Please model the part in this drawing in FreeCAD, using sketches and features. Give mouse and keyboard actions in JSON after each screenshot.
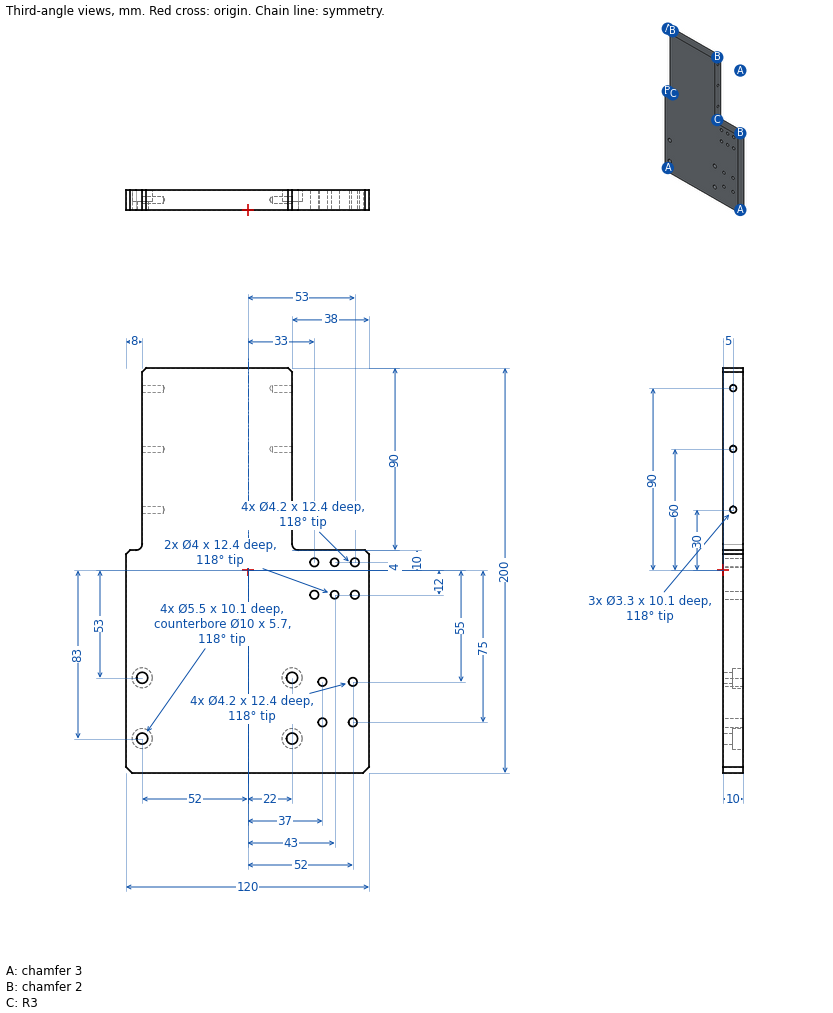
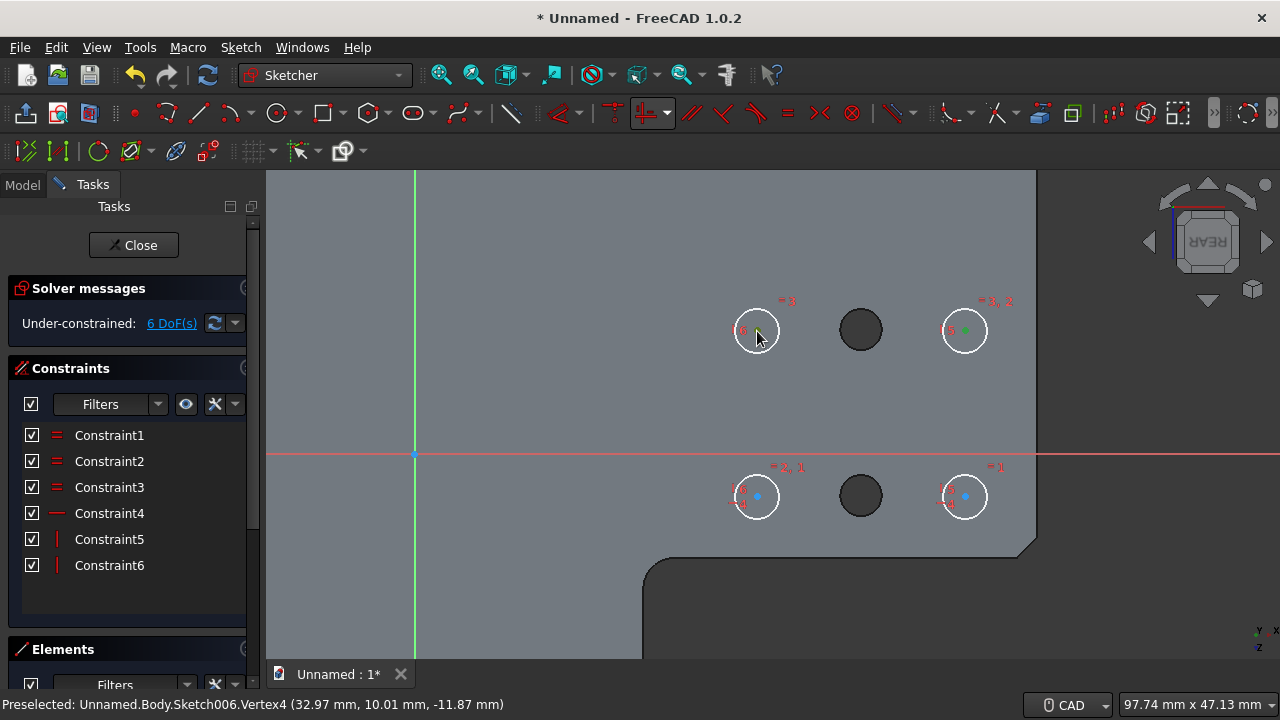
{"action": "left_click", "coordinate": [670, 114]}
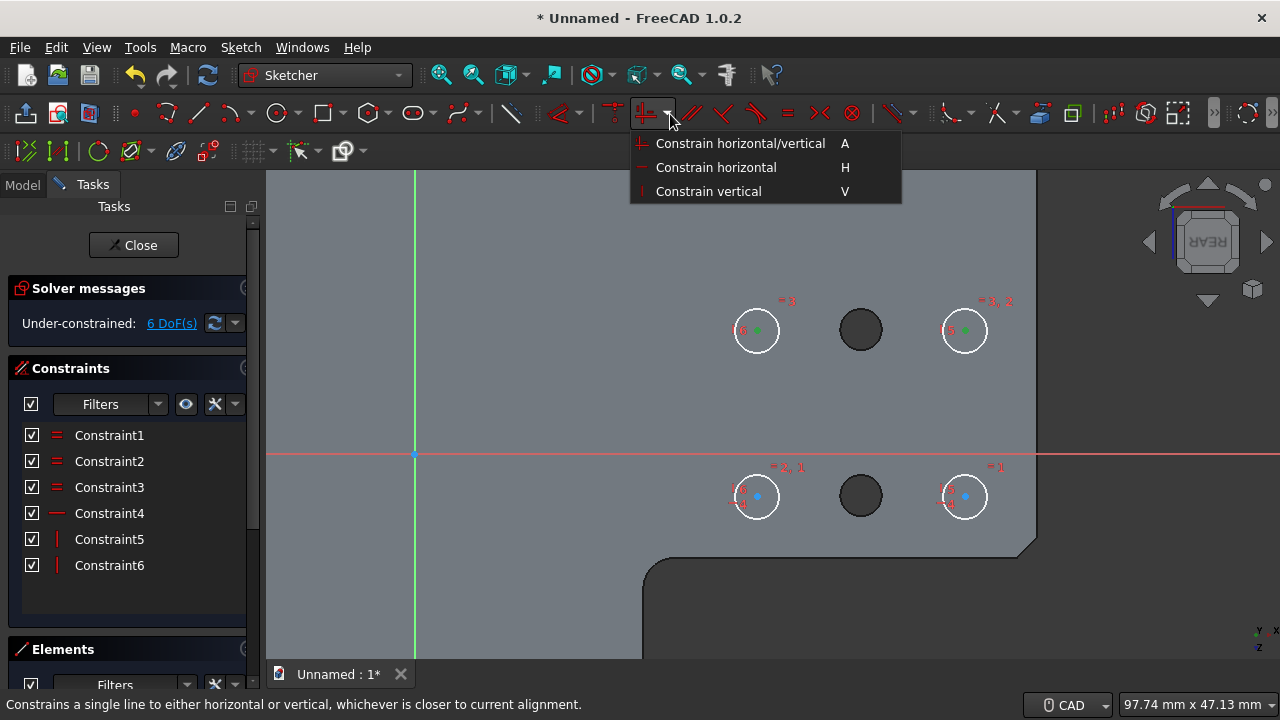
{"action": "left_click", "coordinate": [766, 167]}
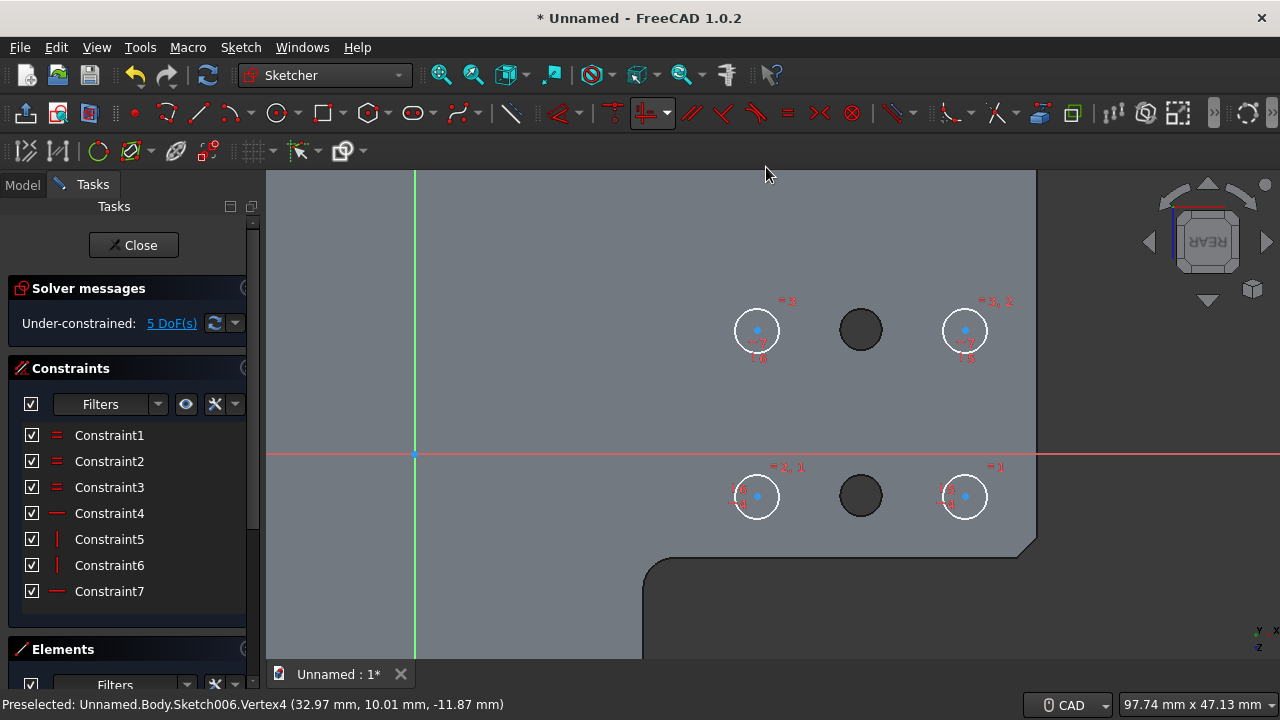
{"action": "key", "text": "d"}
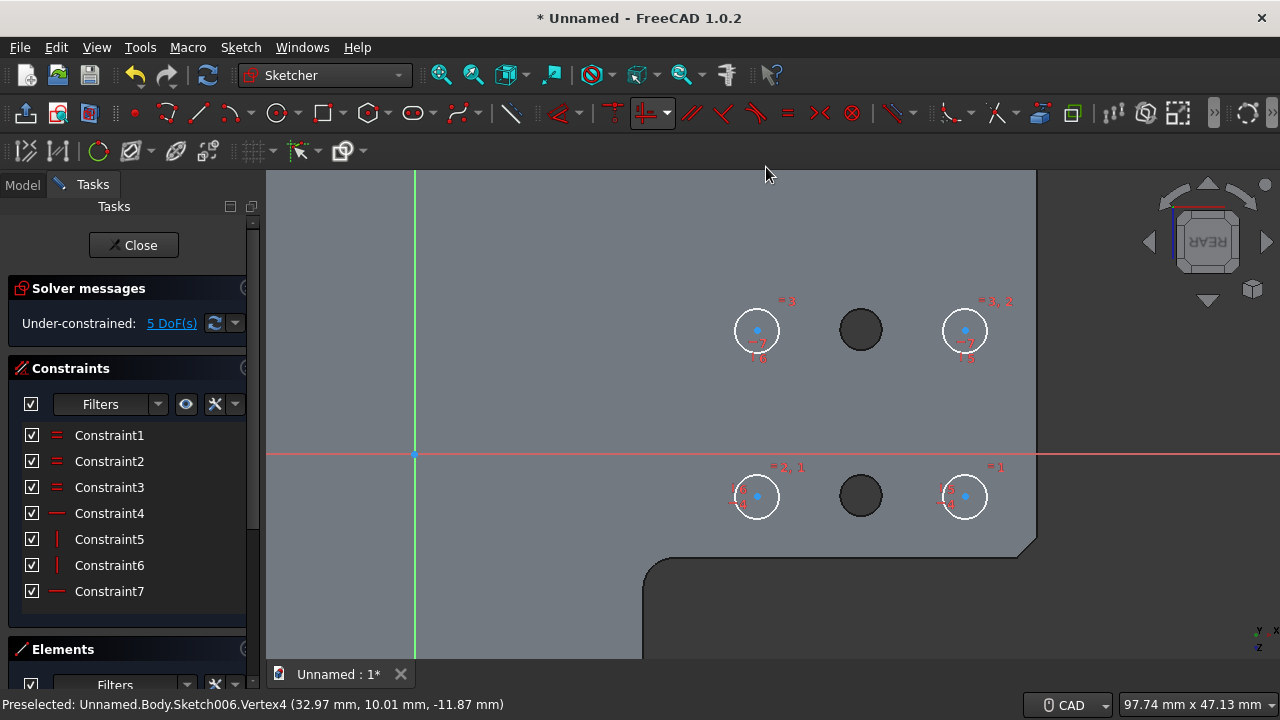
{"action": "left_click", "coordinate": [980, 481]}
{"action": "left_click", "coordinate": [1016, 480]}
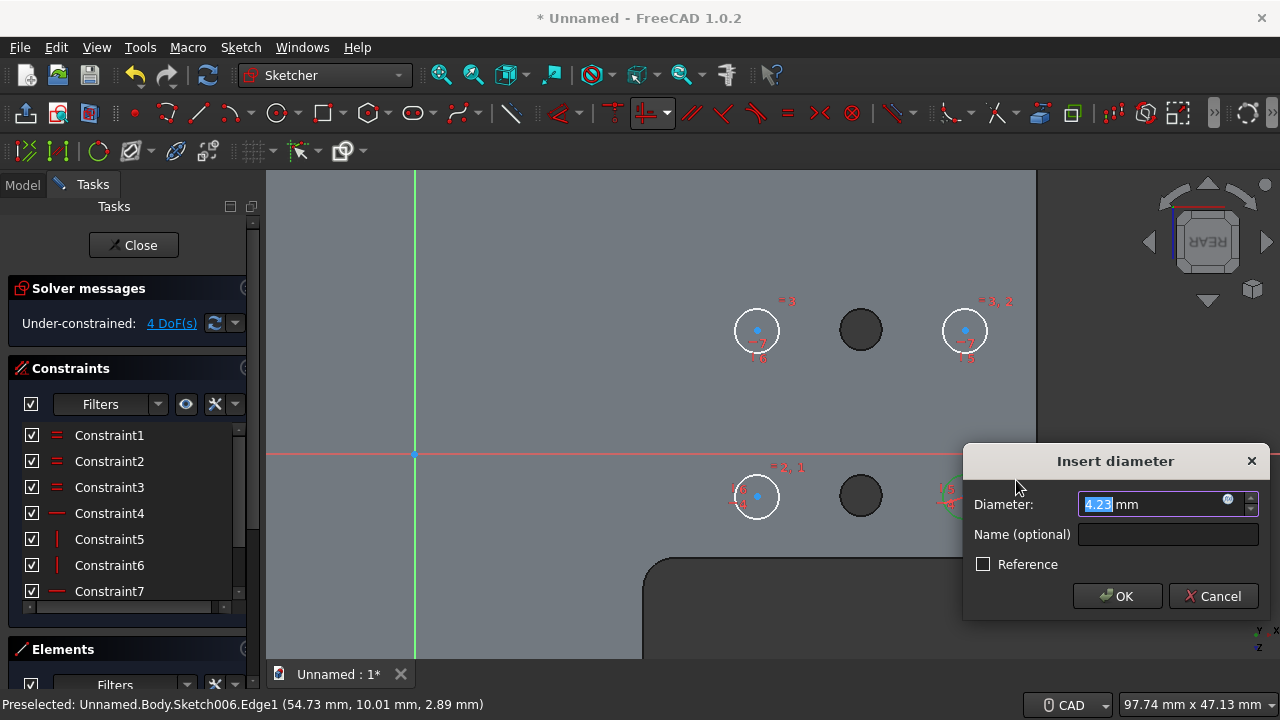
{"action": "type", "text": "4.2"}
{"action": "key", "text": "Return"}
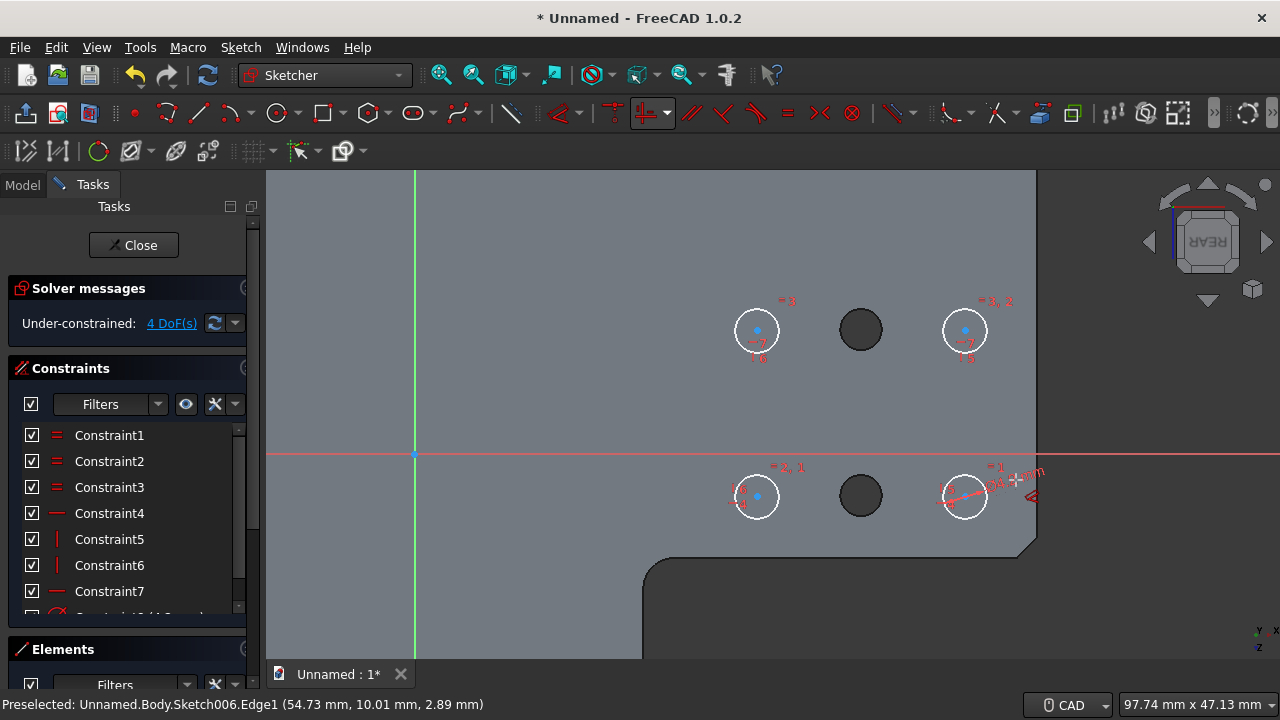
{"action": "left_click", "coordinate": [965, 497]}
{"action": "left_click", "coordinate": [381, 476]}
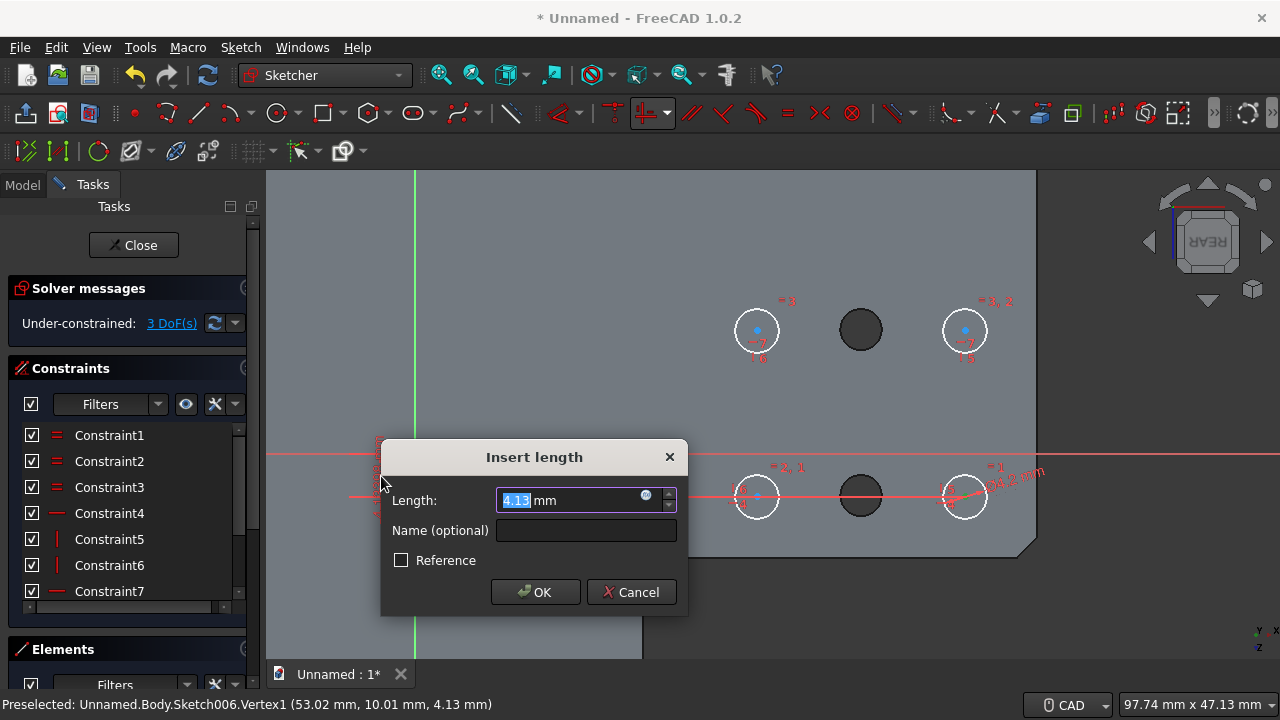
{"action": "type", "text": "4"}
{"action": "key", "text": "Return"}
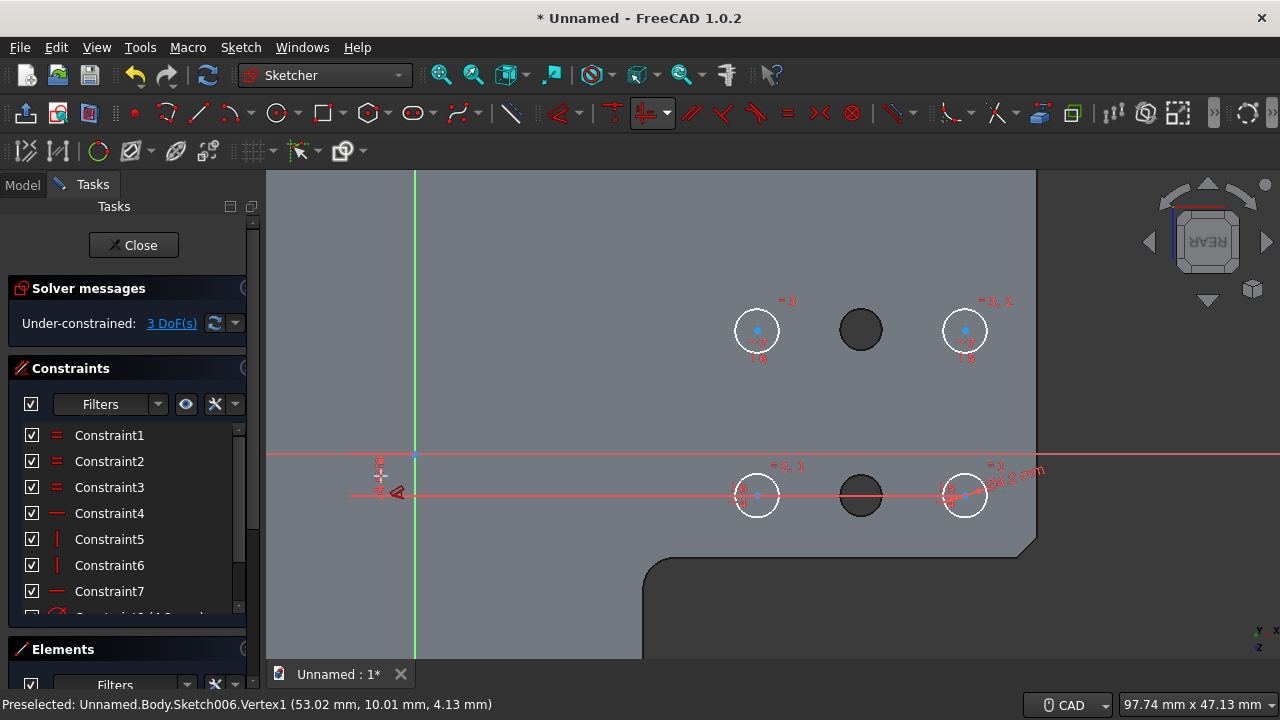
{"action": "left_click", "coordinate": [965, 496]}
{"action": "left_click", "coordinate": [690, 530]}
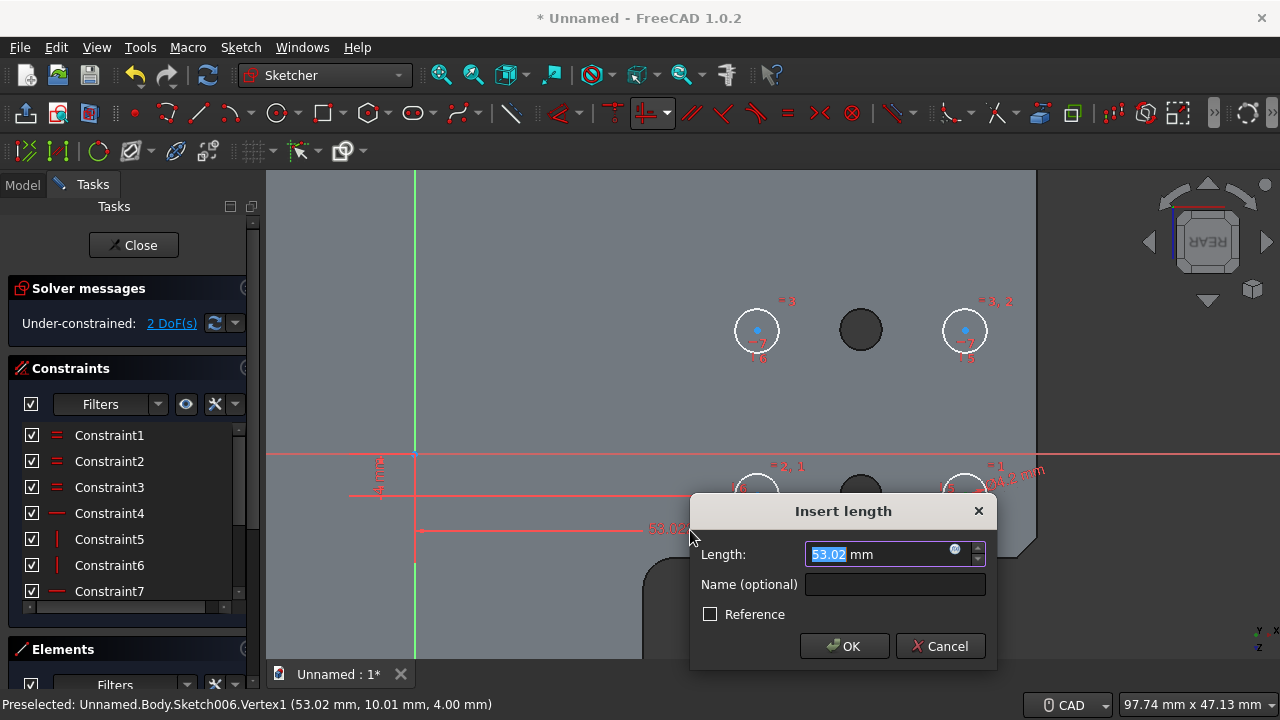
{"action": "type", "text": "53"}
{"action": "key", "text": "Return"}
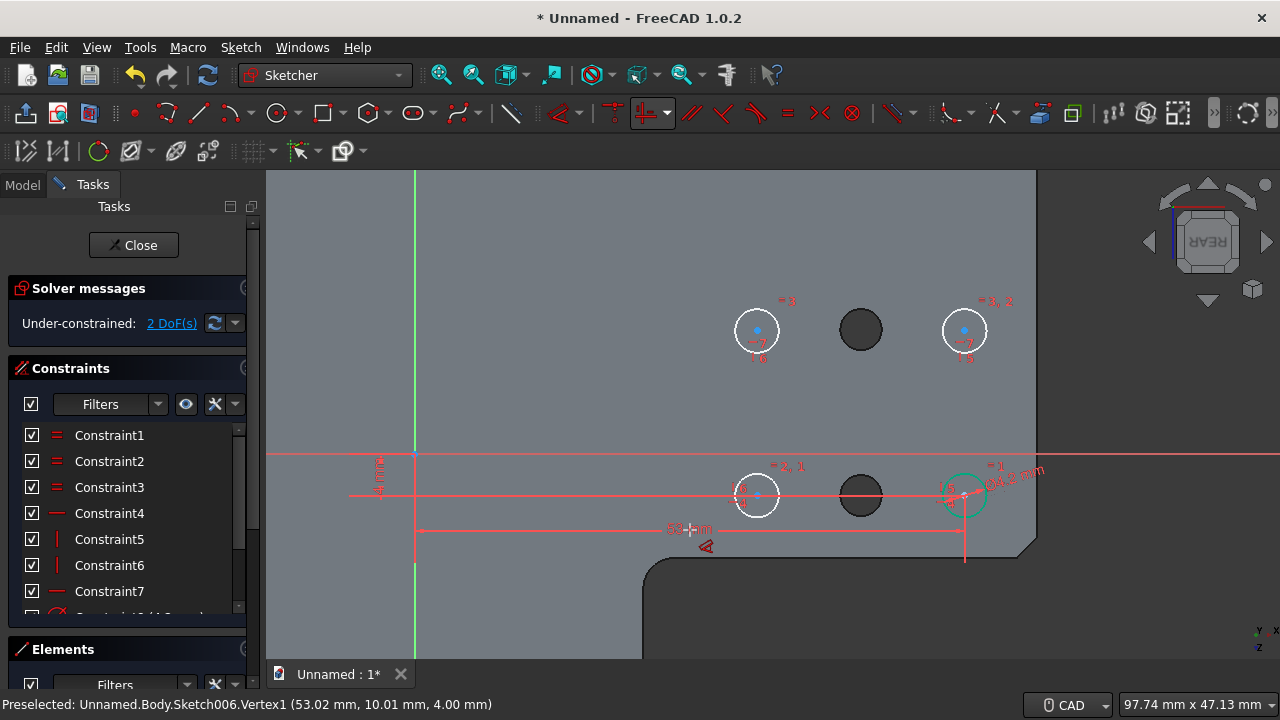
{"action": "left_click", "coordinate": [757, 496]}
{"action": "left_click", "coordinate": [586, 530]}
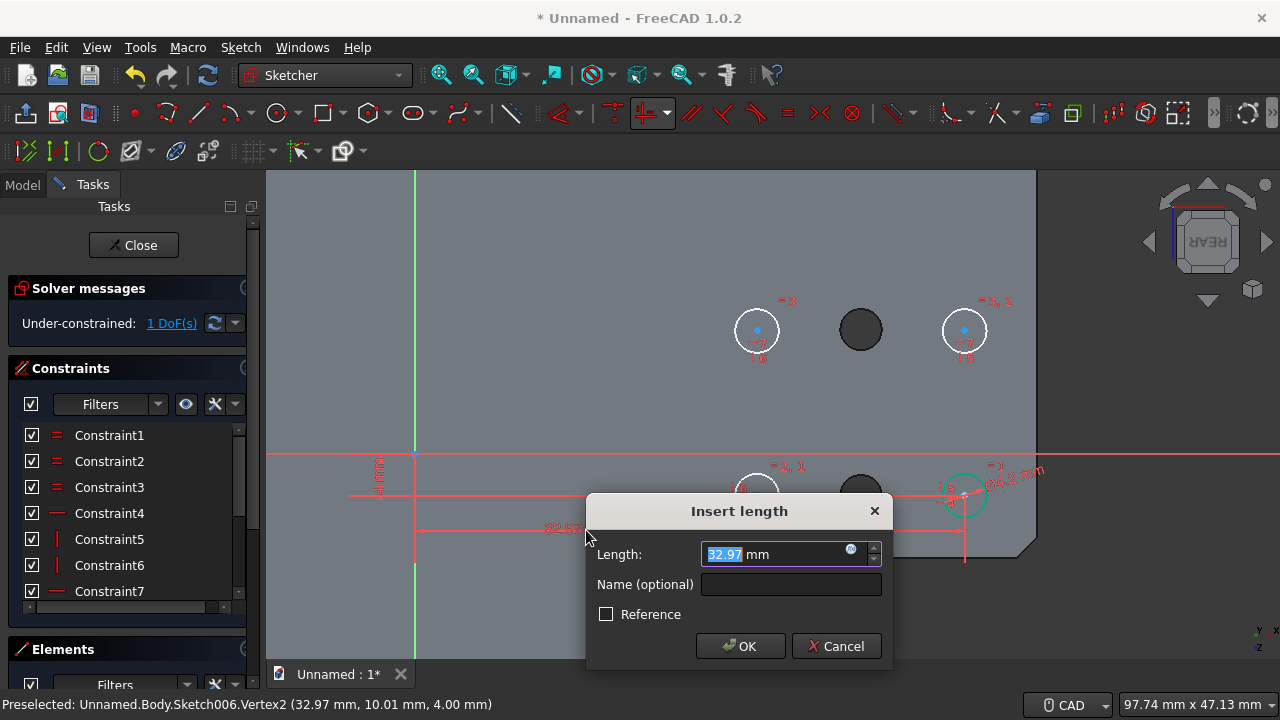
{"action": "type", "text": "33"}
{"action": "key", "text": "Return"}